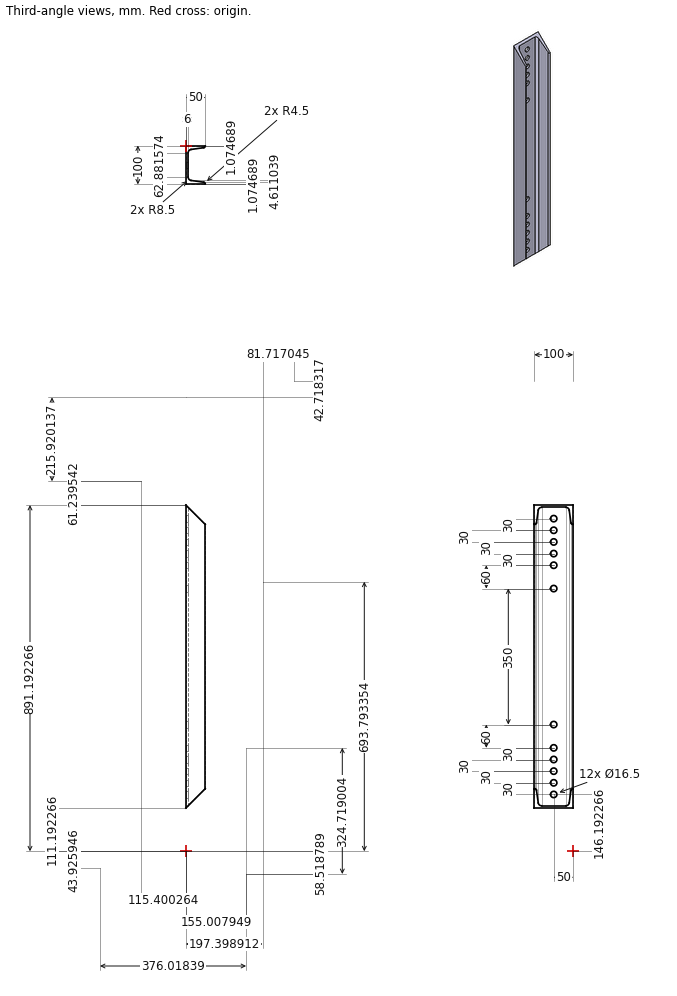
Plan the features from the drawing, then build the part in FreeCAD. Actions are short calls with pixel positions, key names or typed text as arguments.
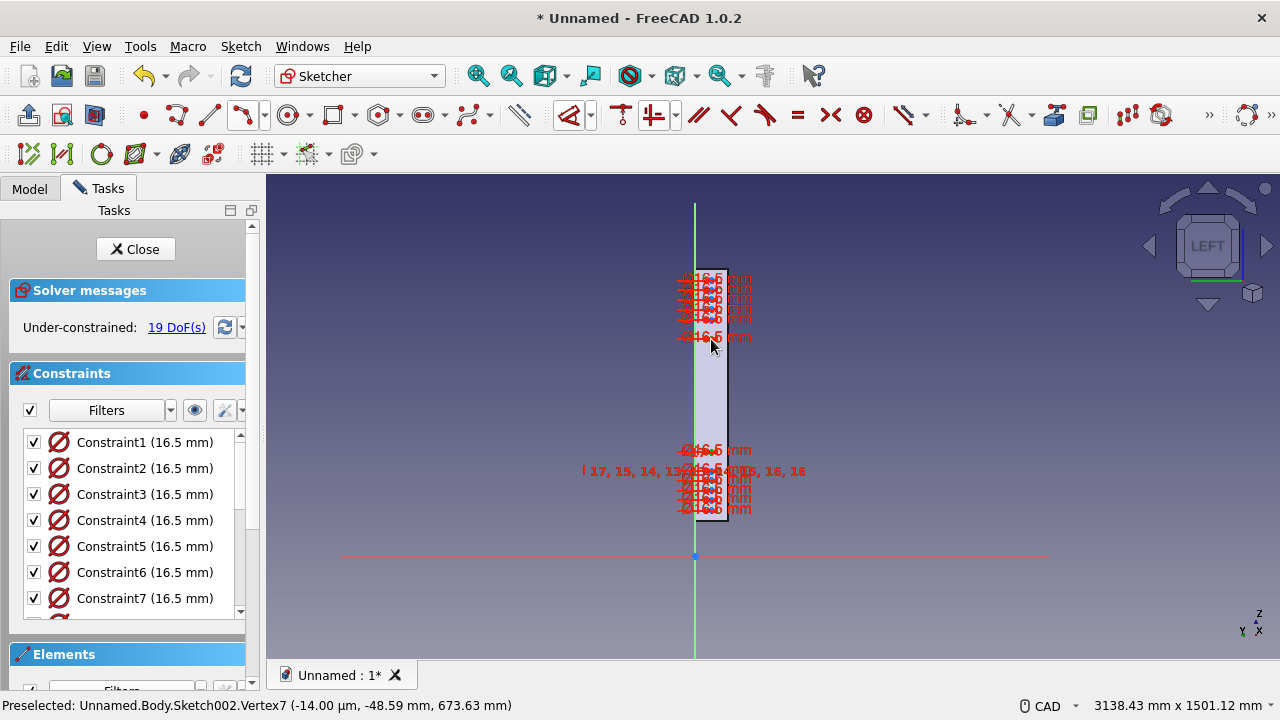
click(676, 116)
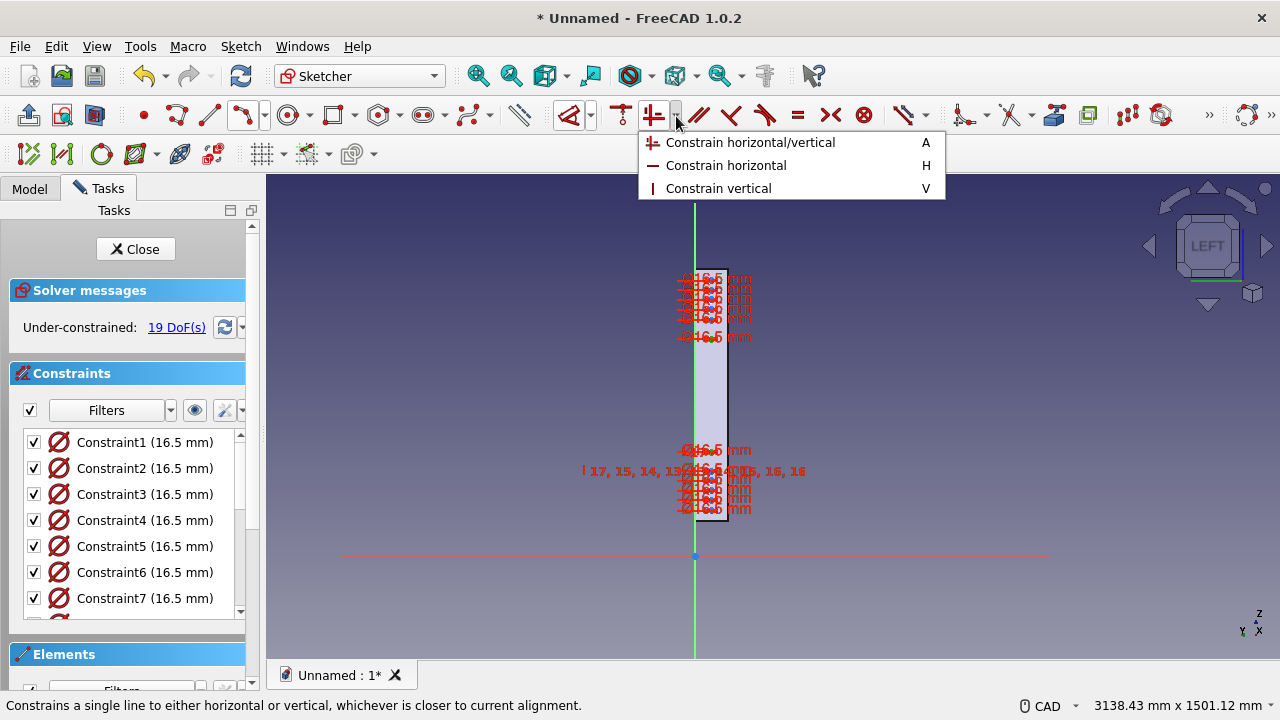
click(792, 188)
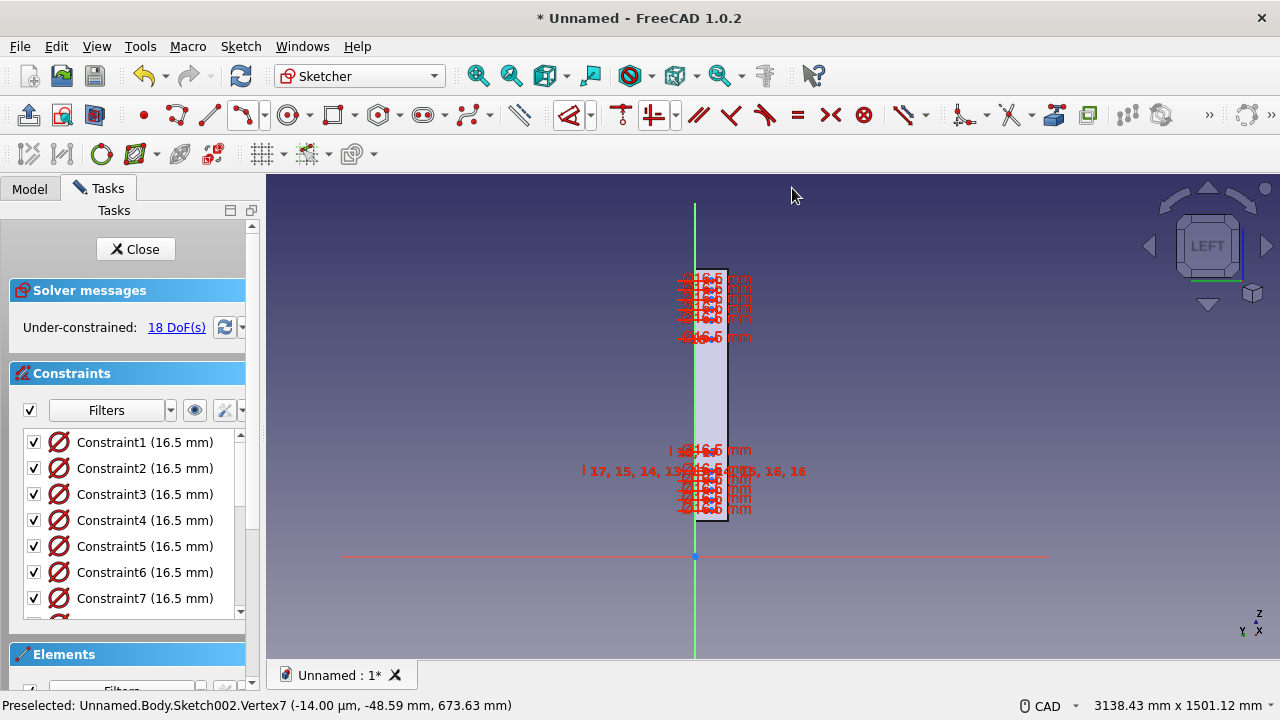
click(711, 339)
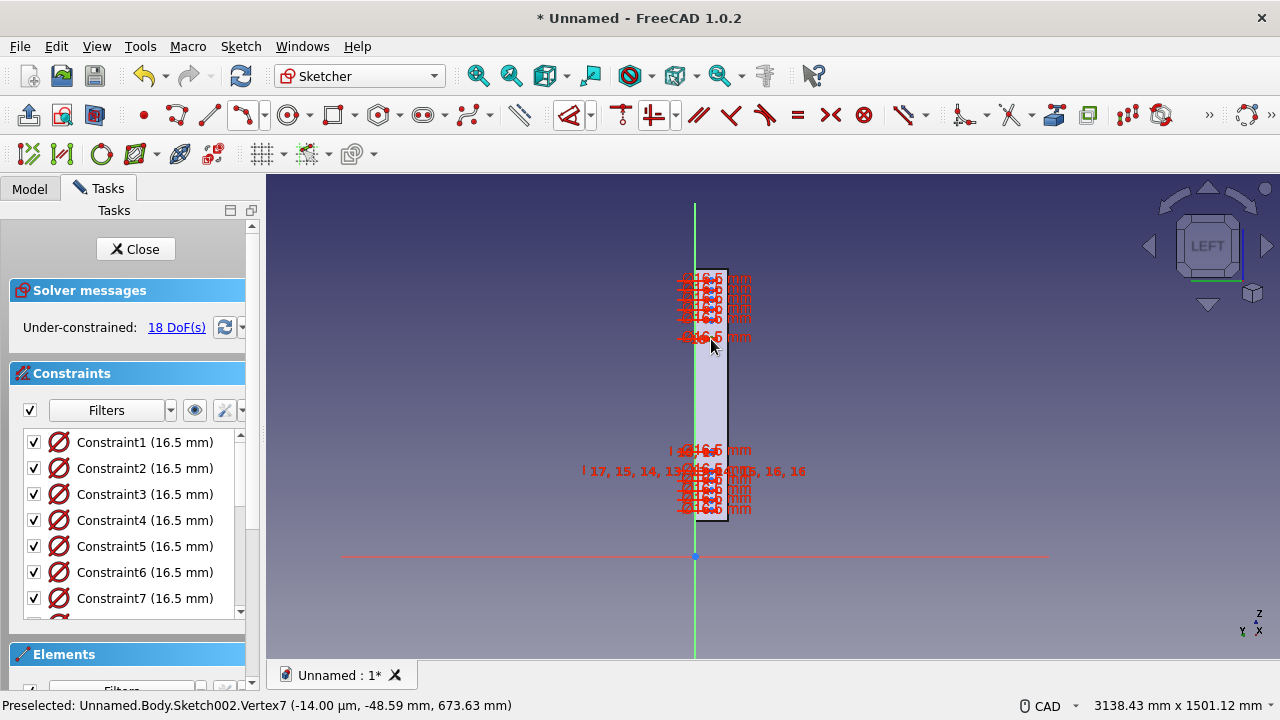
click(711, 320)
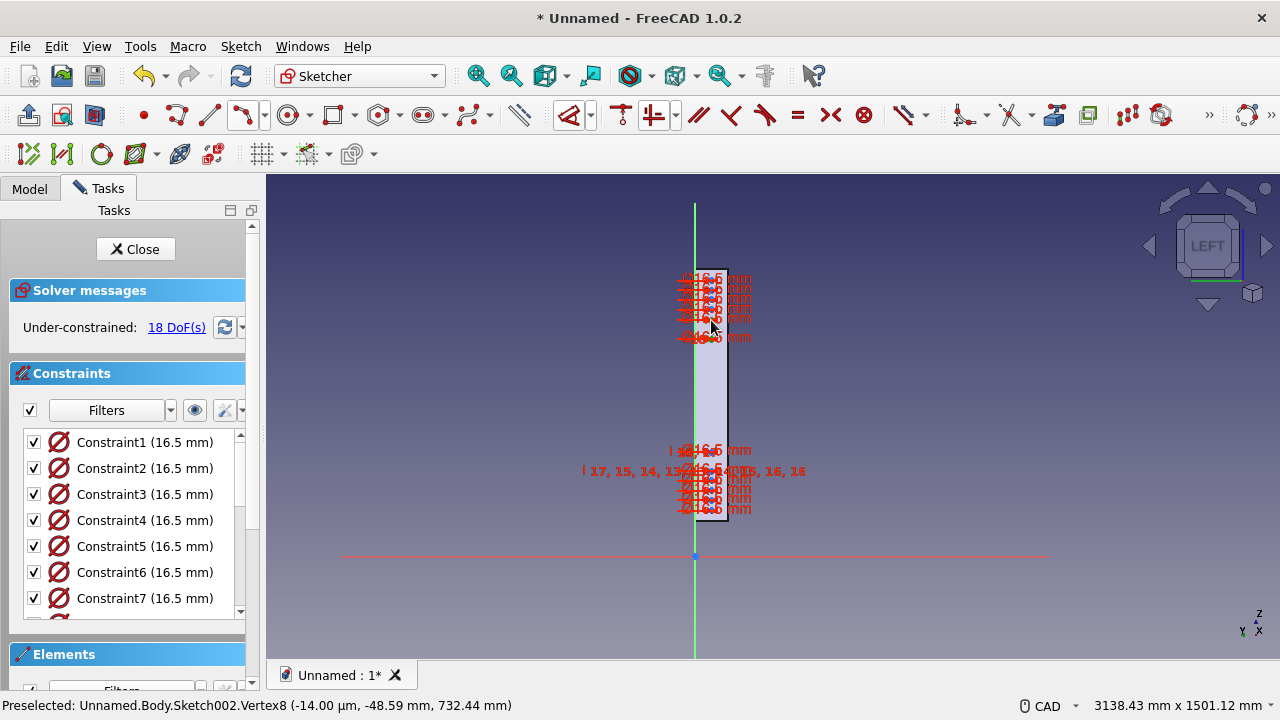
click(676, 116)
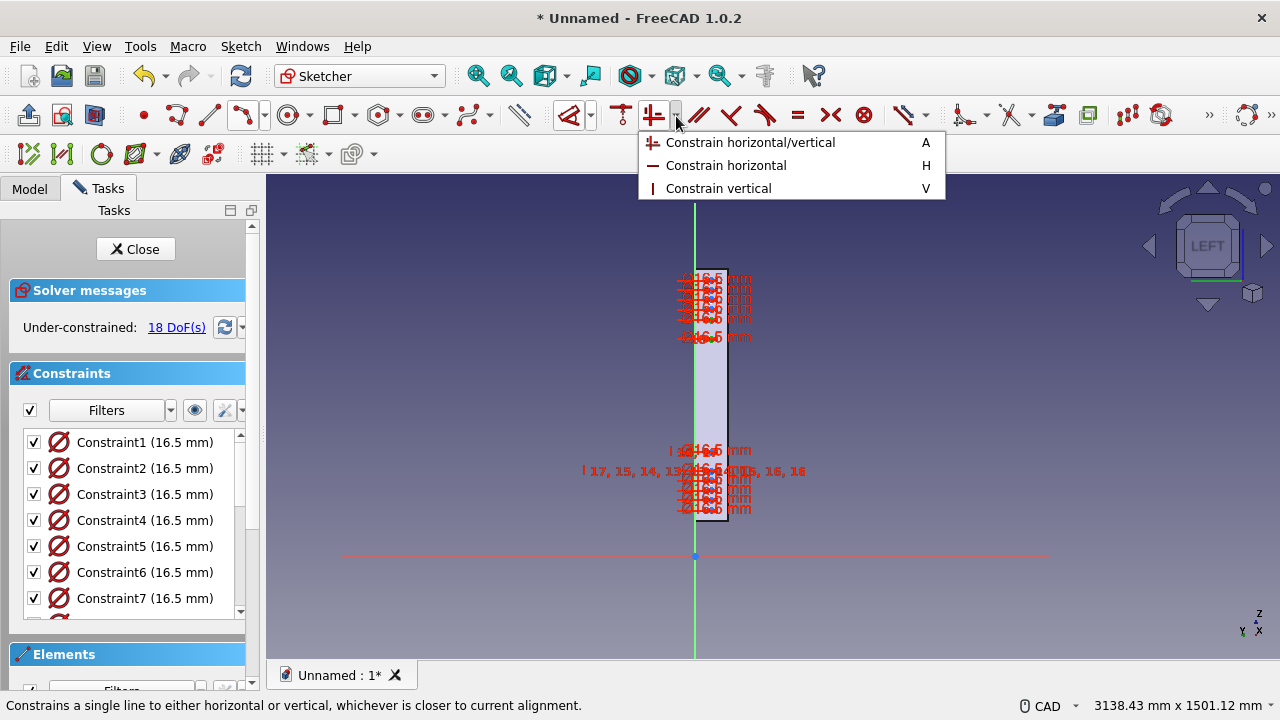
click(792, 188)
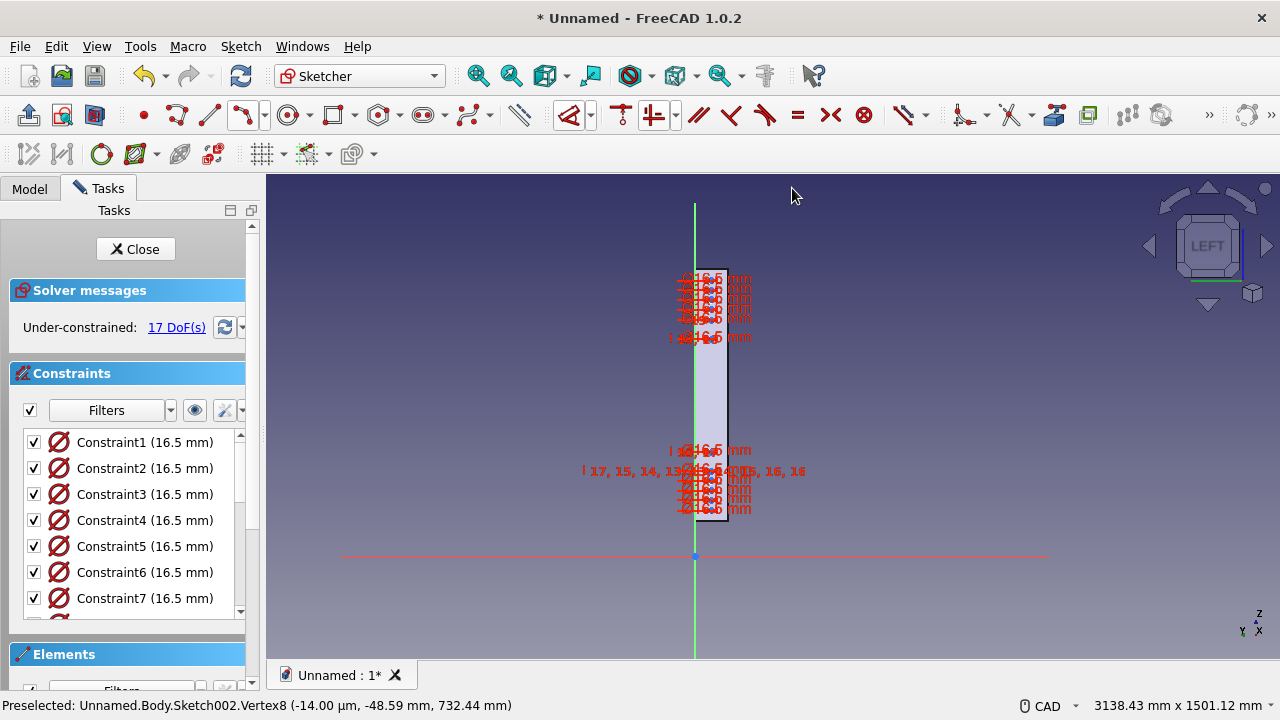
click(711, 320)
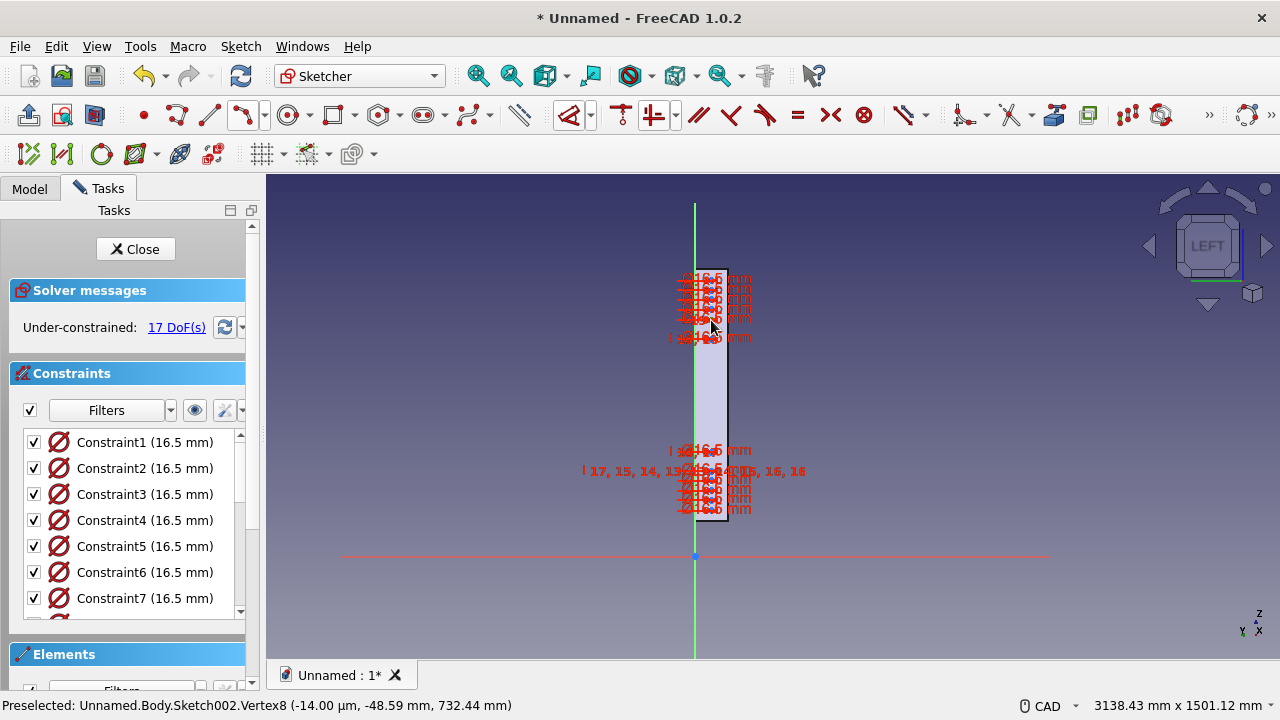
scroll(711, 310, up, 2)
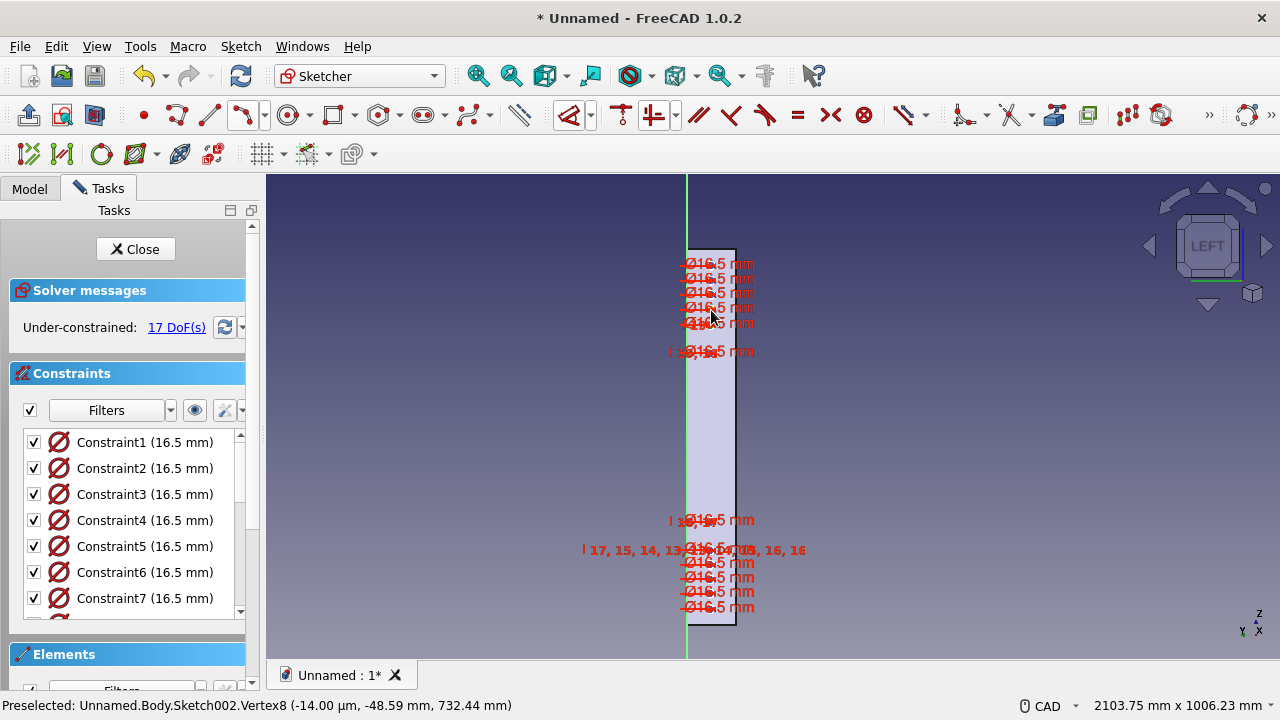
click(711, 310)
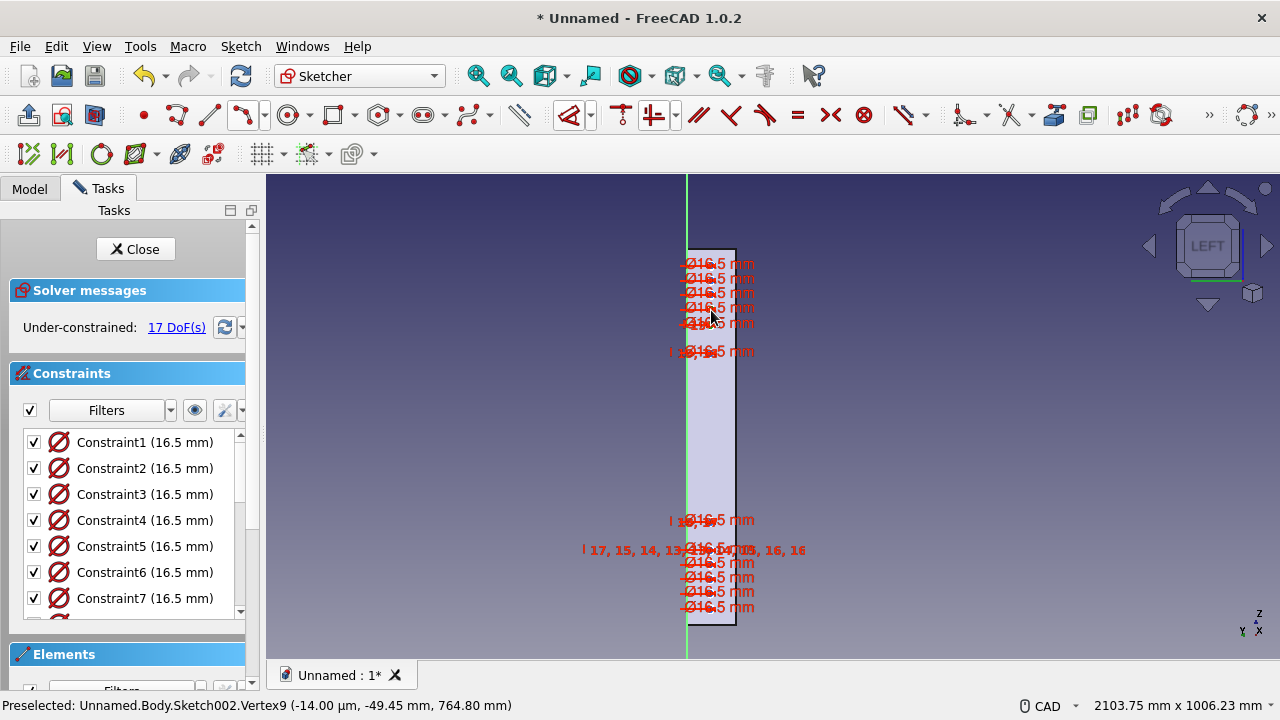
click(676, 116)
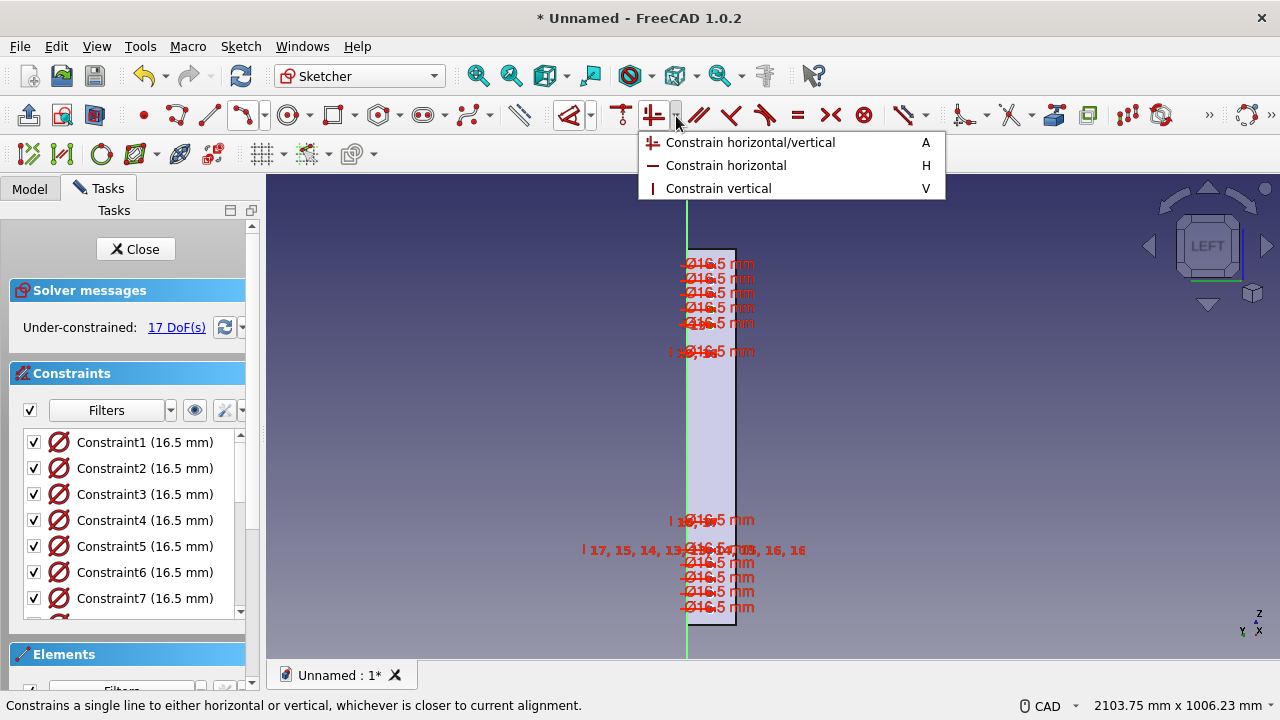
click(792, 188)